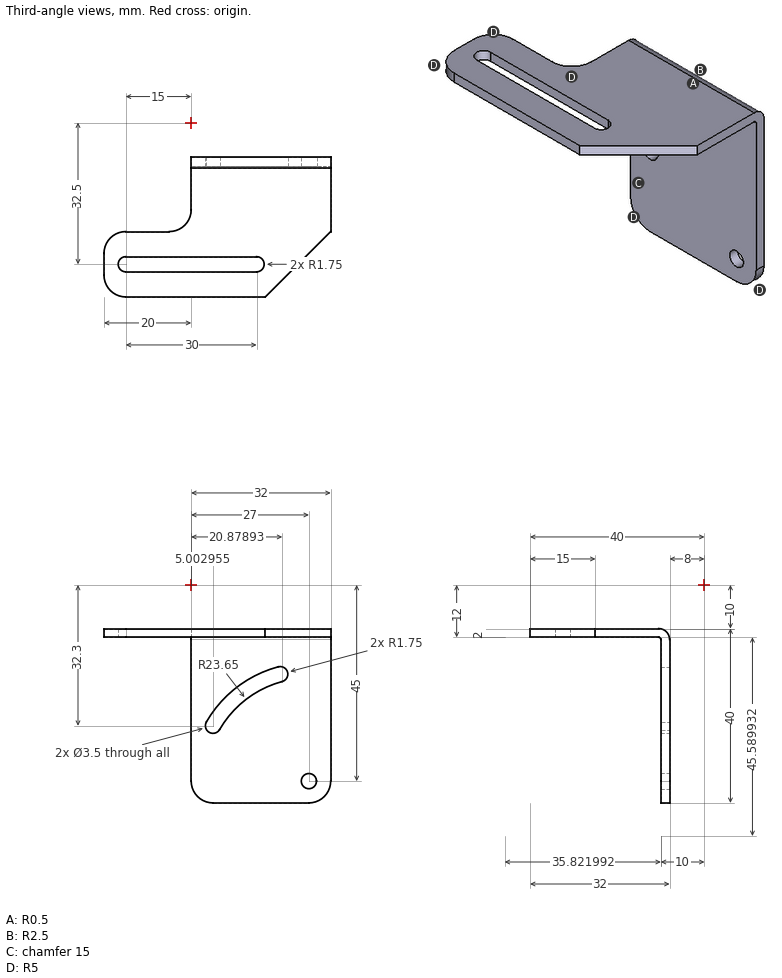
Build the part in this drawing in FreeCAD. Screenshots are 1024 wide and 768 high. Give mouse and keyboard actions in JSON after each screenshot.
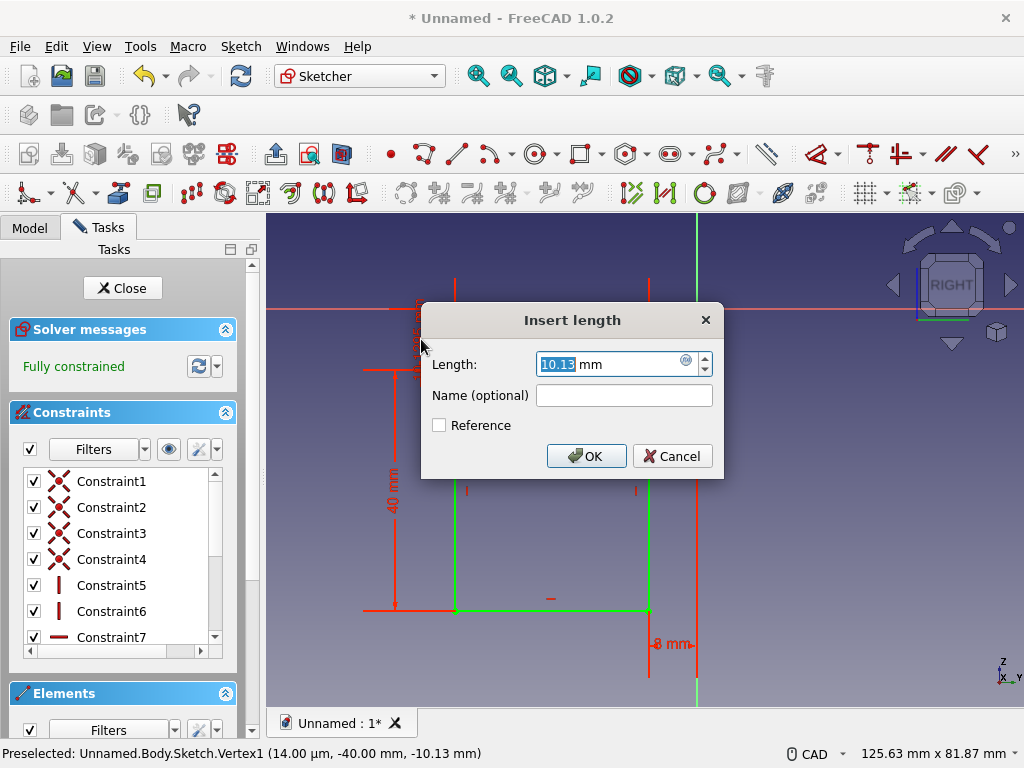
{"action": "type", "text": "10"}
{"action": "key", "text": "Return"}
{"action": "key", "text": "Escape"}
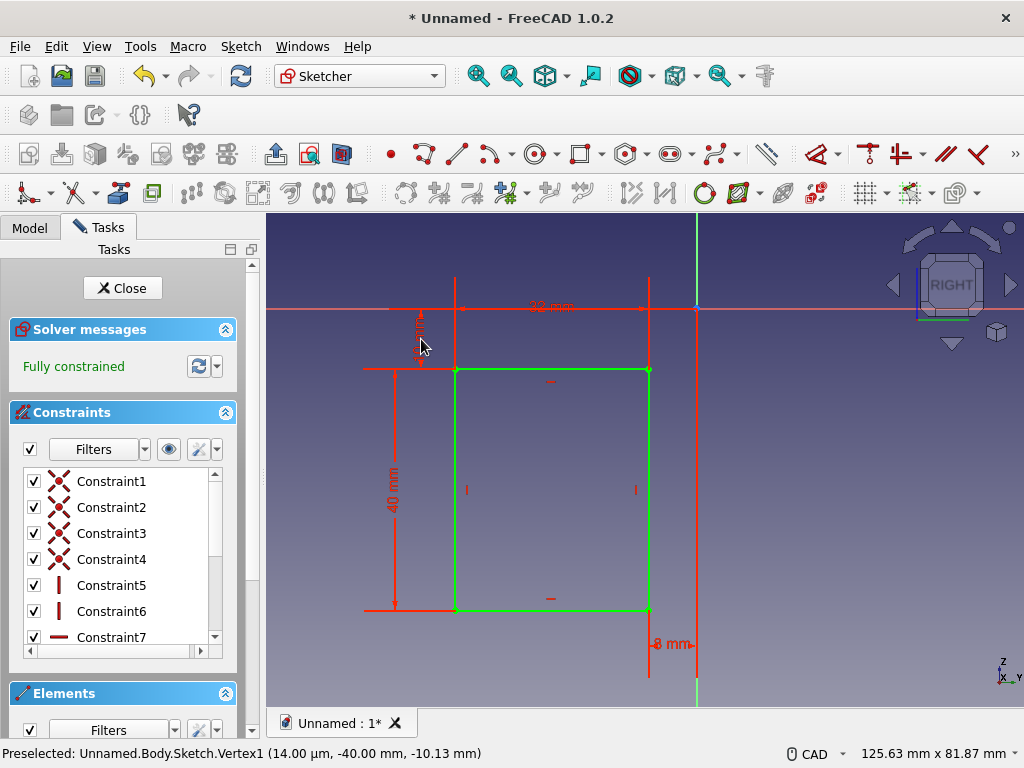
{"action": "left_click", "coordinate": [123, 288]}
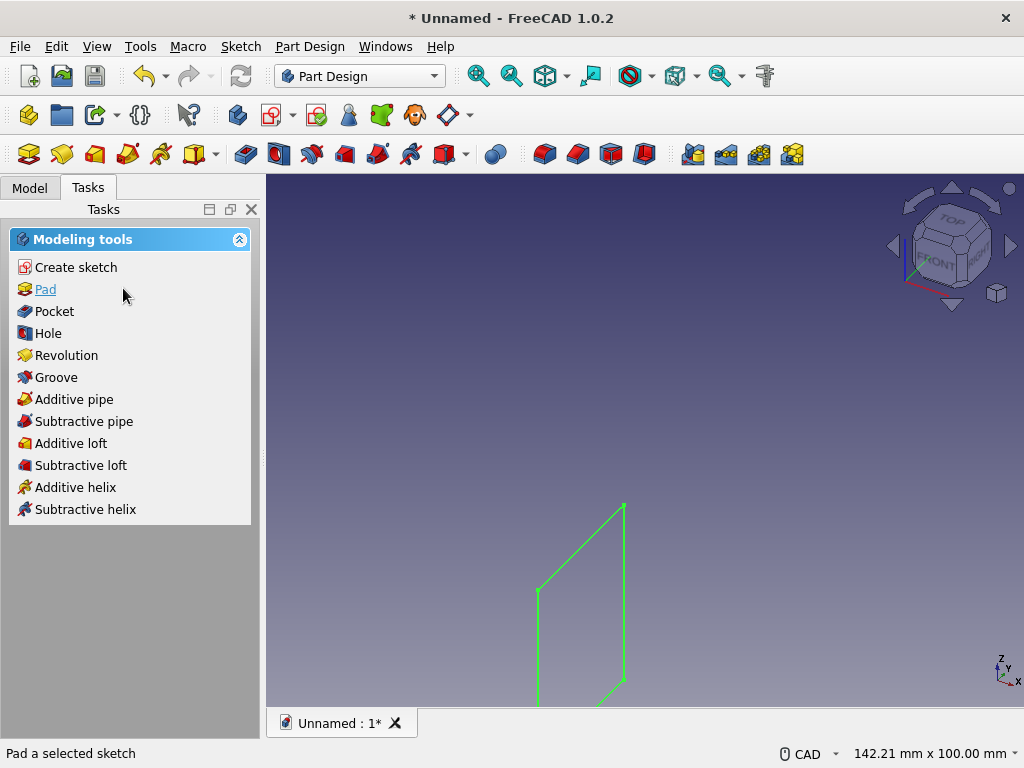
{"action": "left_click", "coordinate": [29, 154]}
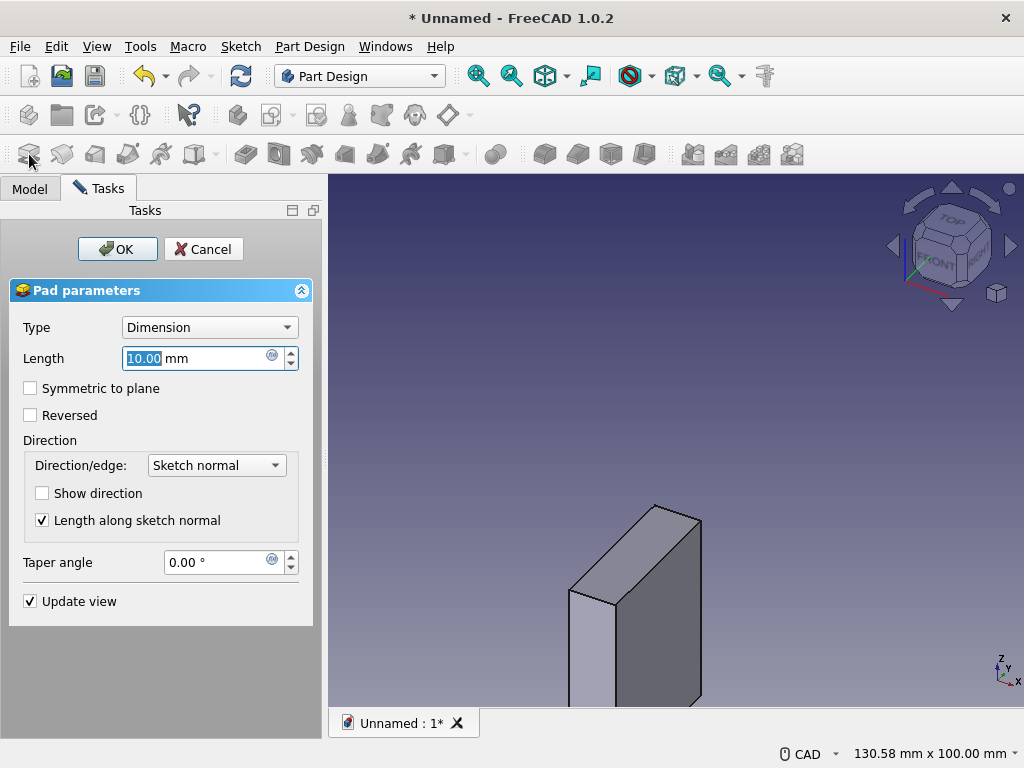
{"action": "type", "text": "32"}
{"action": "key", "text": "Tab"}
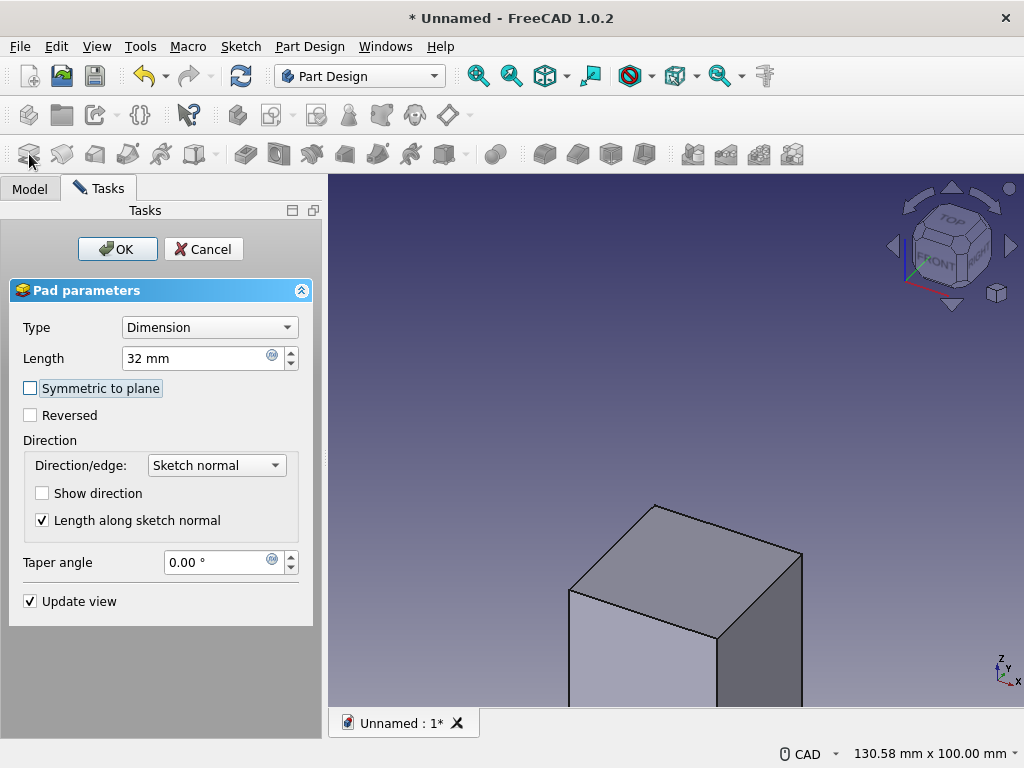
{"action": "left_click", "coordinate": [118, 249]}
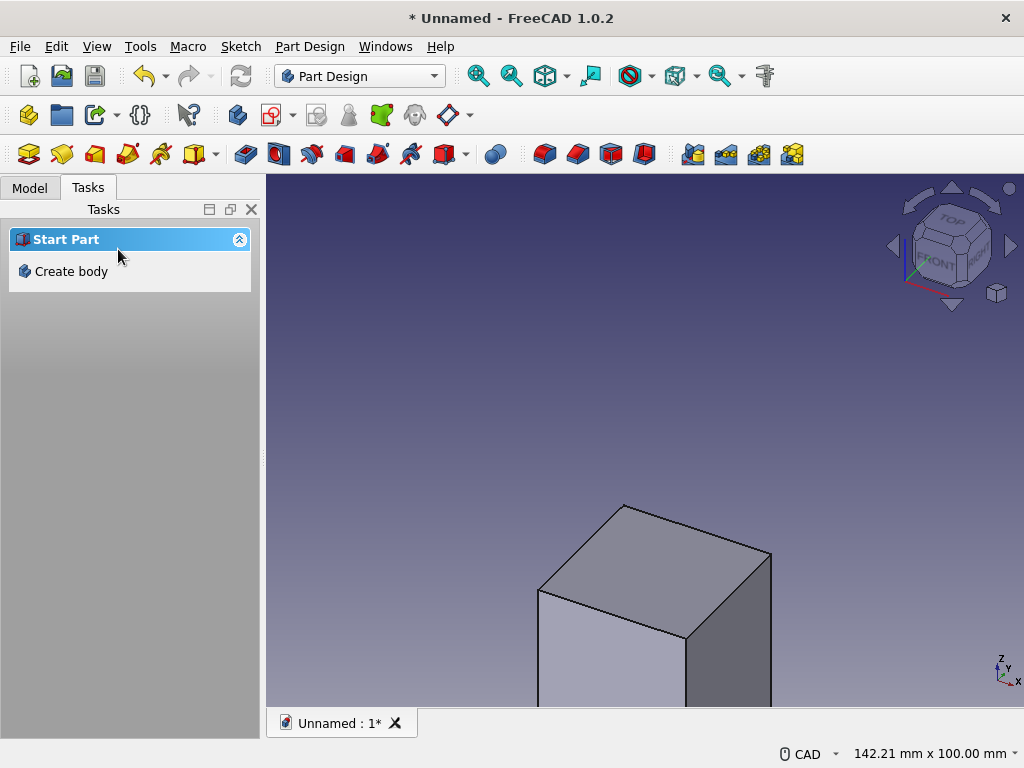
{"action": "key", "text": "v f"}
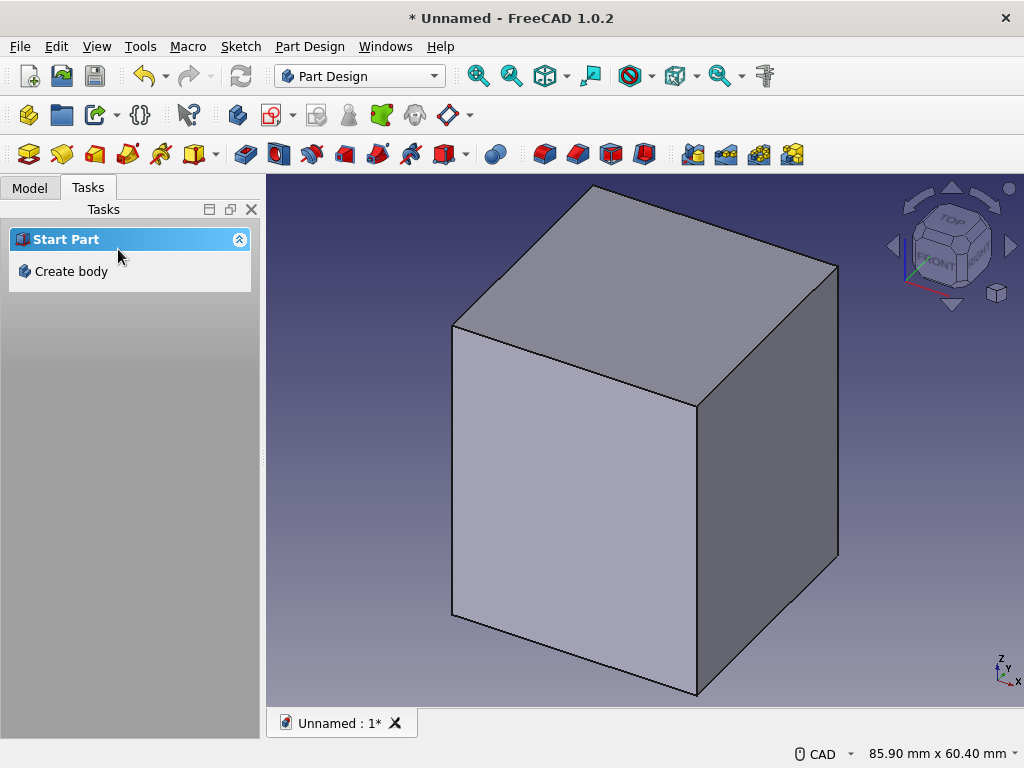
{"action": "left_click", "coordinate": [767, 480]}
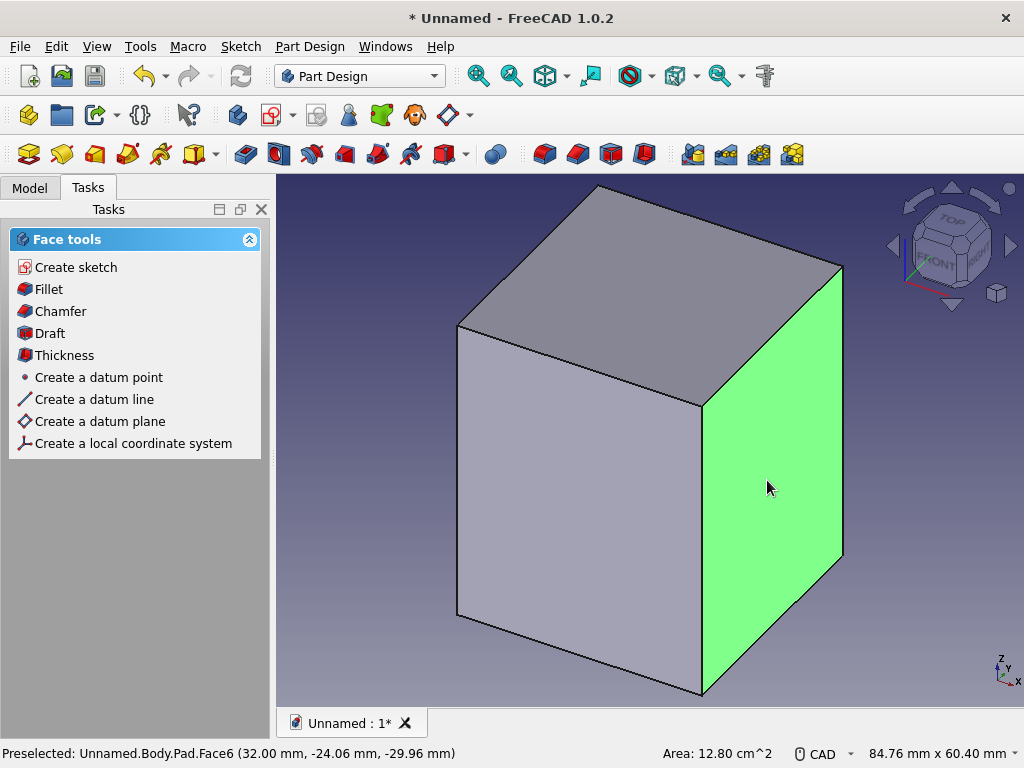
{"action": "left_click", "coordinate": [270, 116]}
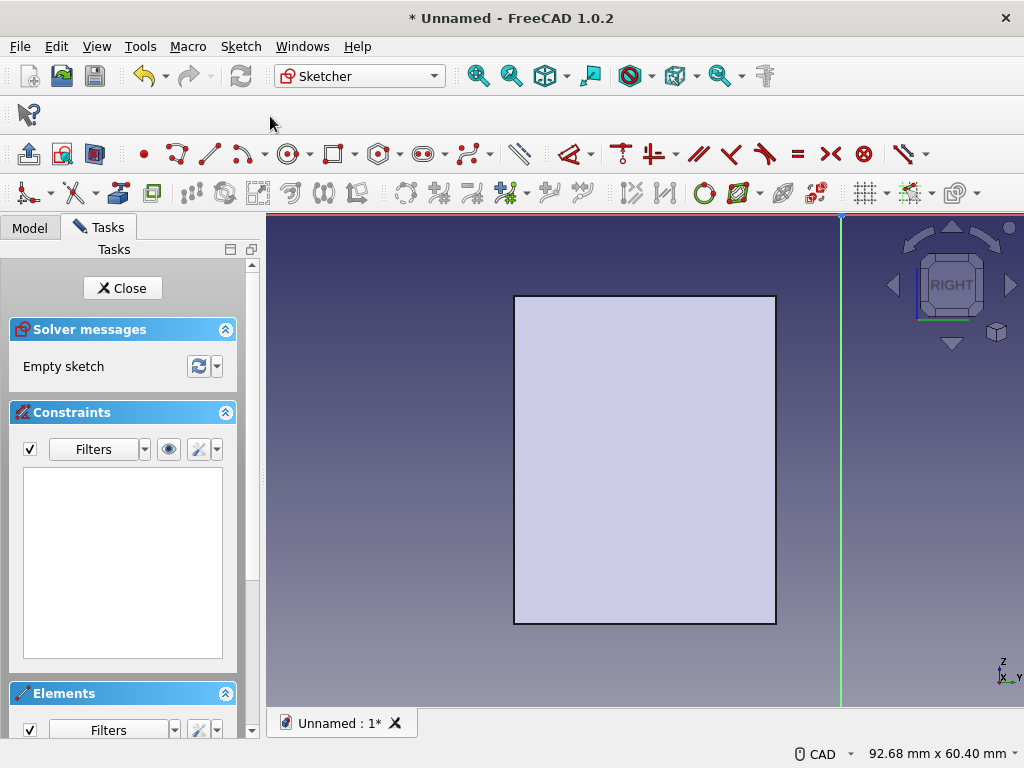
{"action": "scroll", "coordinate": [419, 480], "scroll_direction": "down", "scroll_amount": 2}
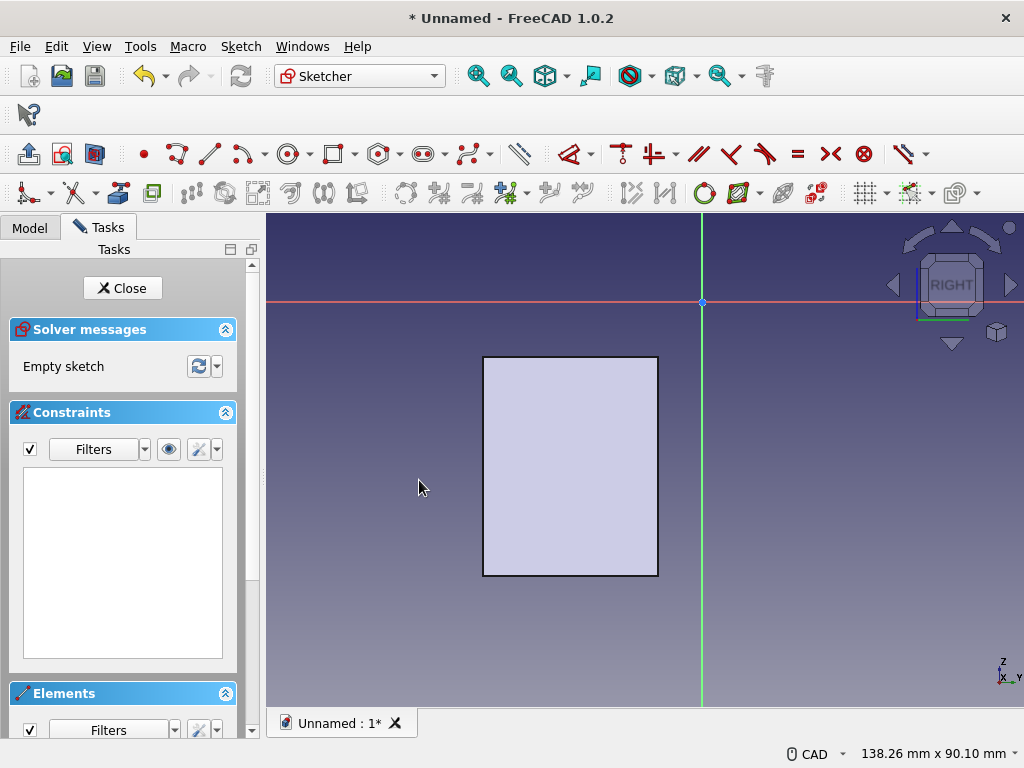
{"action": "key", "text": "g r"}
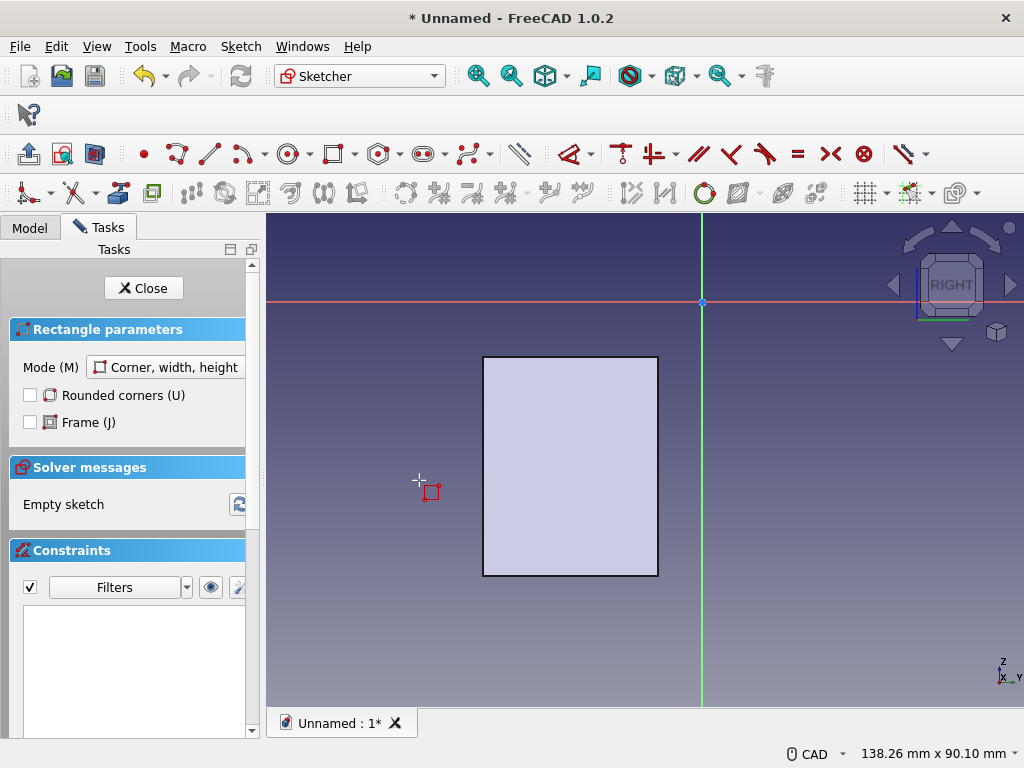
{"action": "left_click", "coordinate": [451, 368]}
{"action": "mouse_move", "coordinate": [647, 618]}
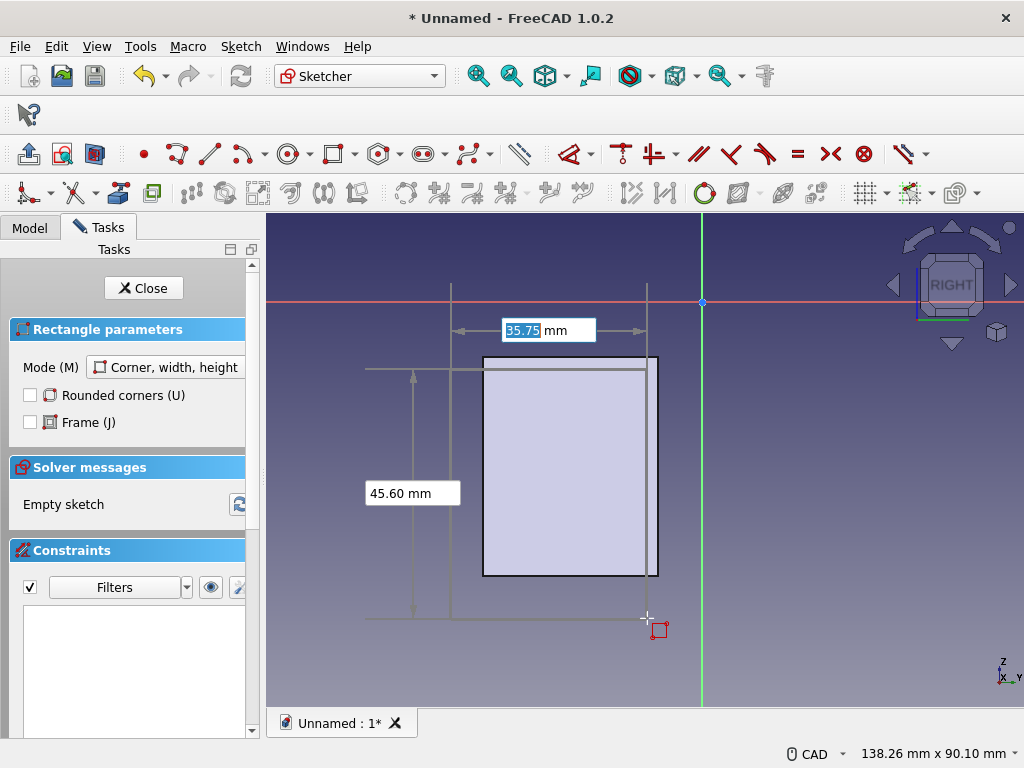
{"action": "type", "text": "35.821992"}
{"action": "key", "text": "Tab"}
{"action": "type", "text": "45.589932"}
{"action": "key", "text": "Return"}
{"action": "key", "text": "Escape"}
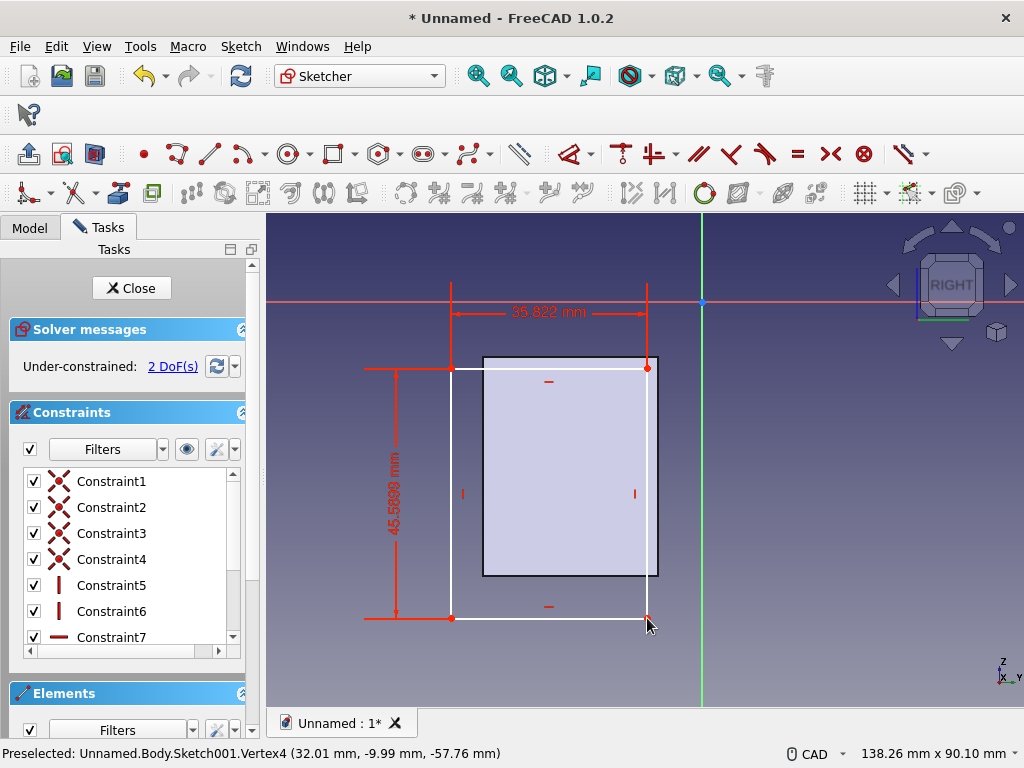
{"action": "key", "text": "d"}